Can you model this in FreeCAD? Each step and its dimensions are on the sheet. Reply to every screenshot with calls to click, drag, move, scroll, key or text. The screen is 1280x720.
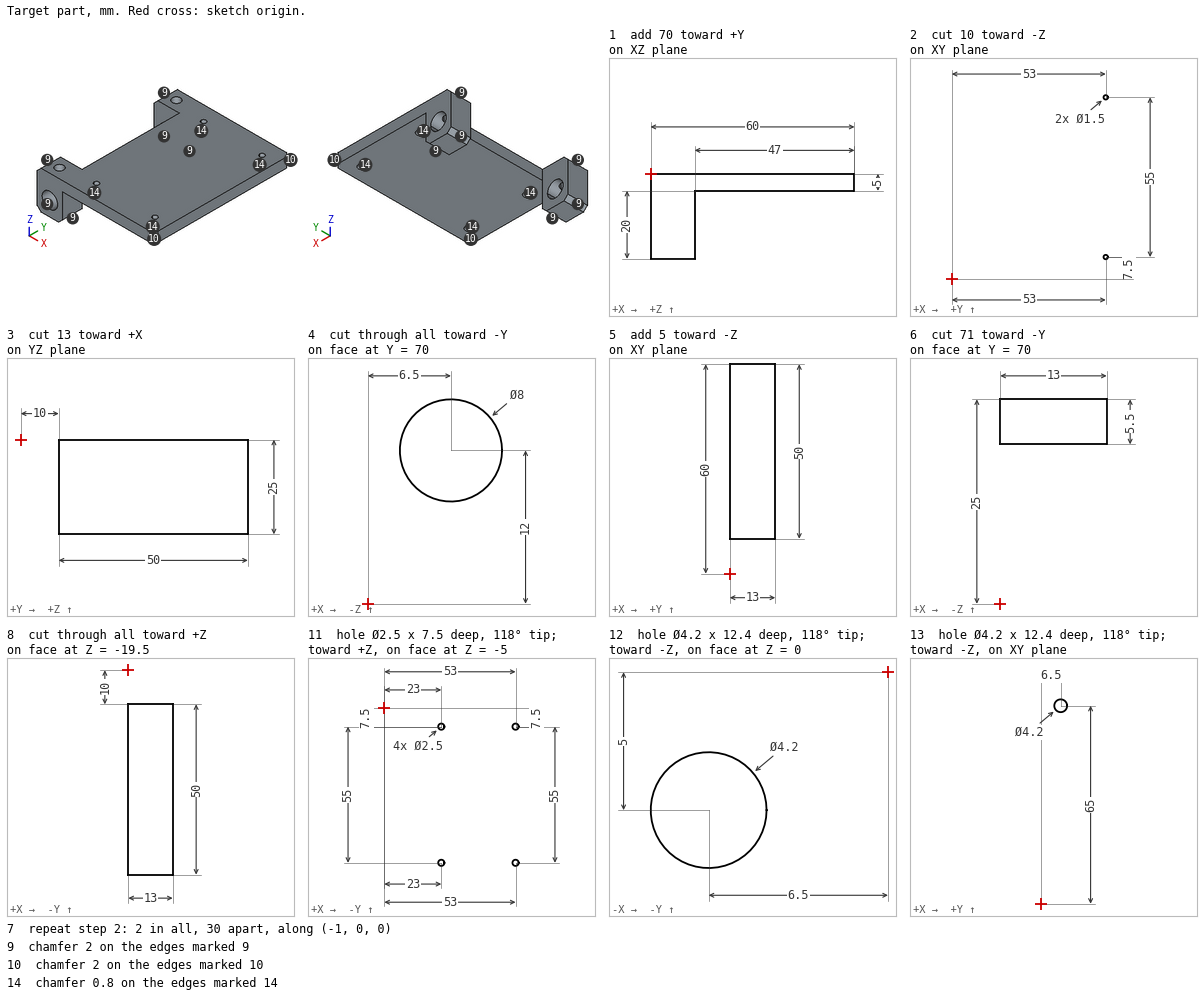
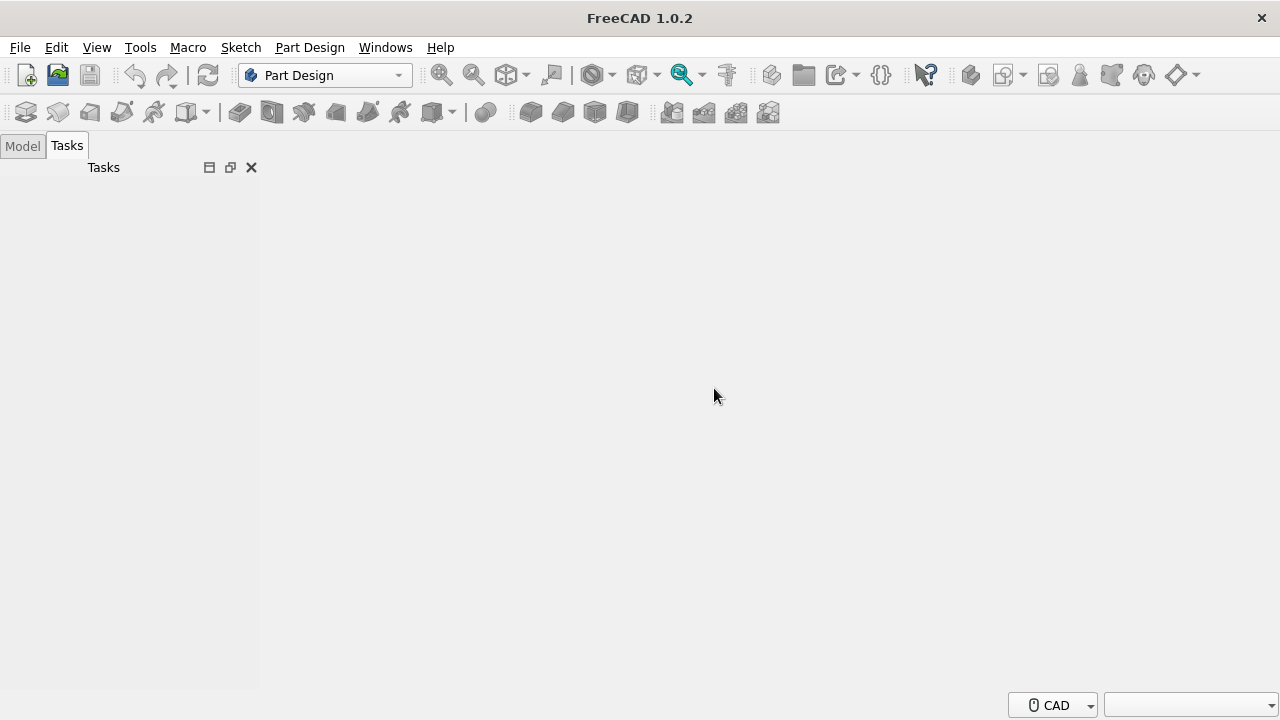
click(26, 76)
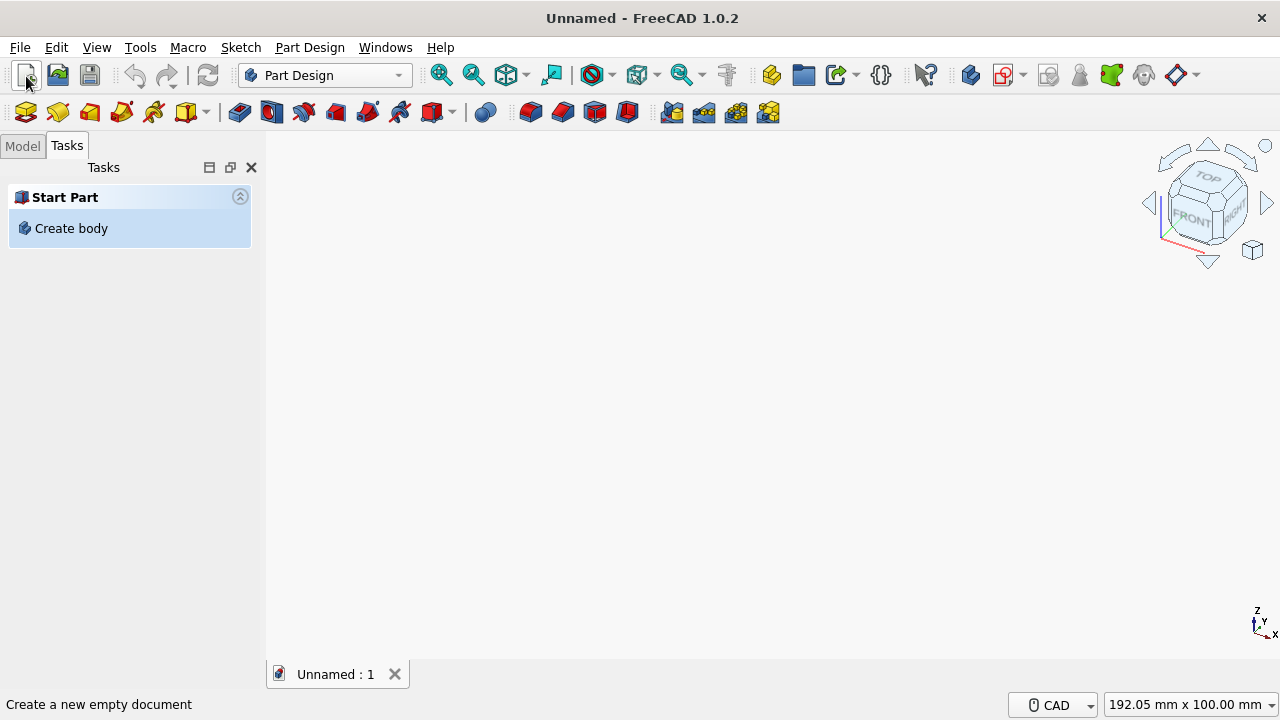
click(1004, 76)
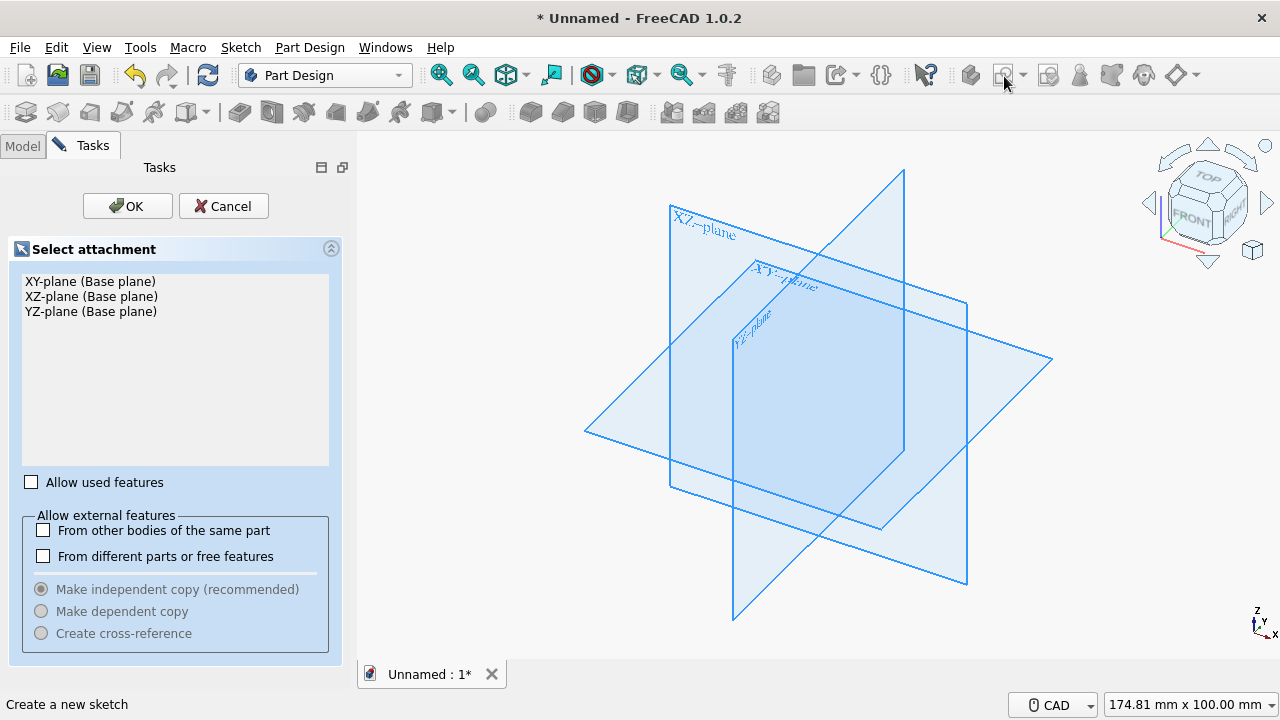
click(82, 296)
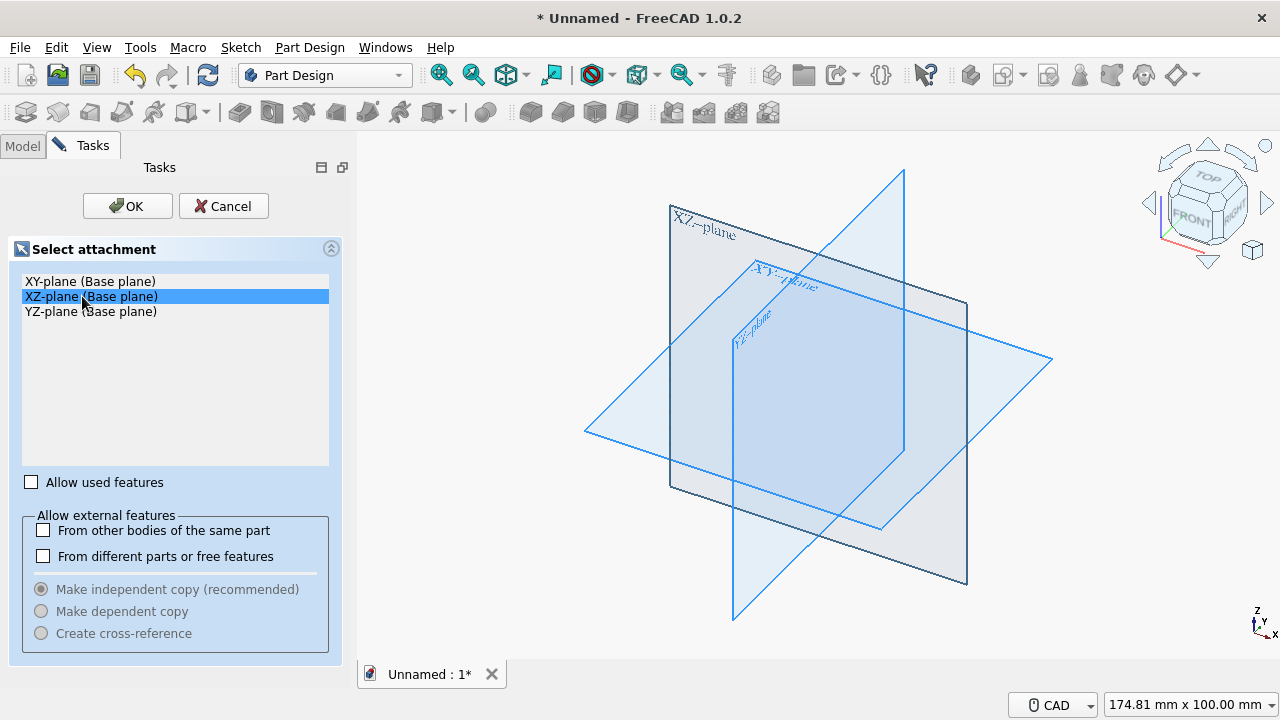
click(128, 206)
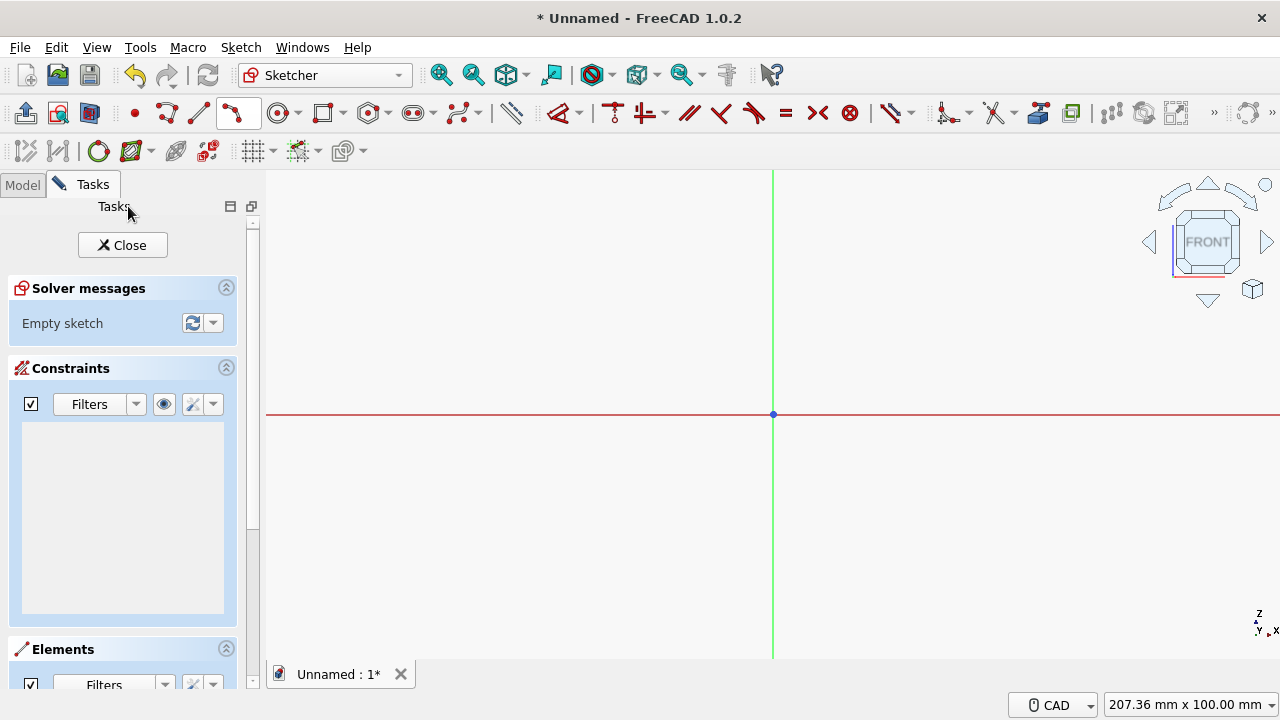
scroll(1115, 550, up, 3)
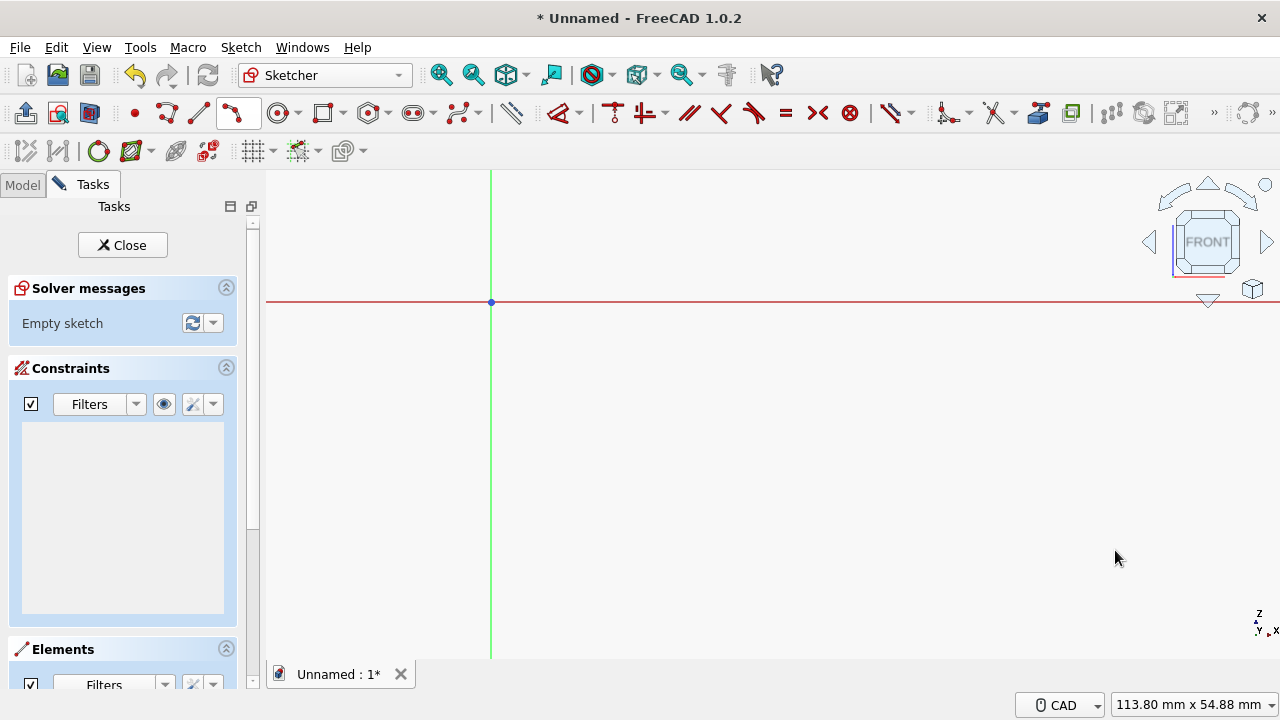
key(g)
key(m)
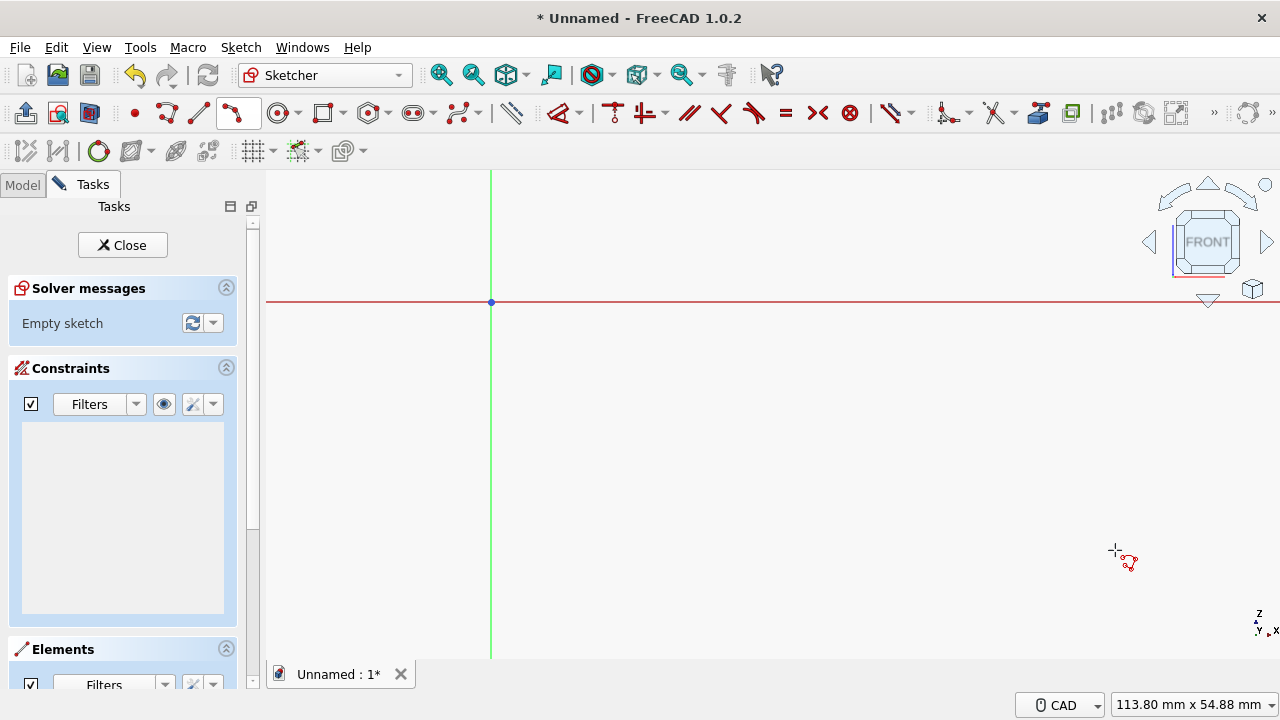
click(491, 302)
click(1026, 311)
click(1026, 347)
click(607, 347)
click(607, 525)
click(500, 525)
click(491, 302)
key(Escape)
key(Escape)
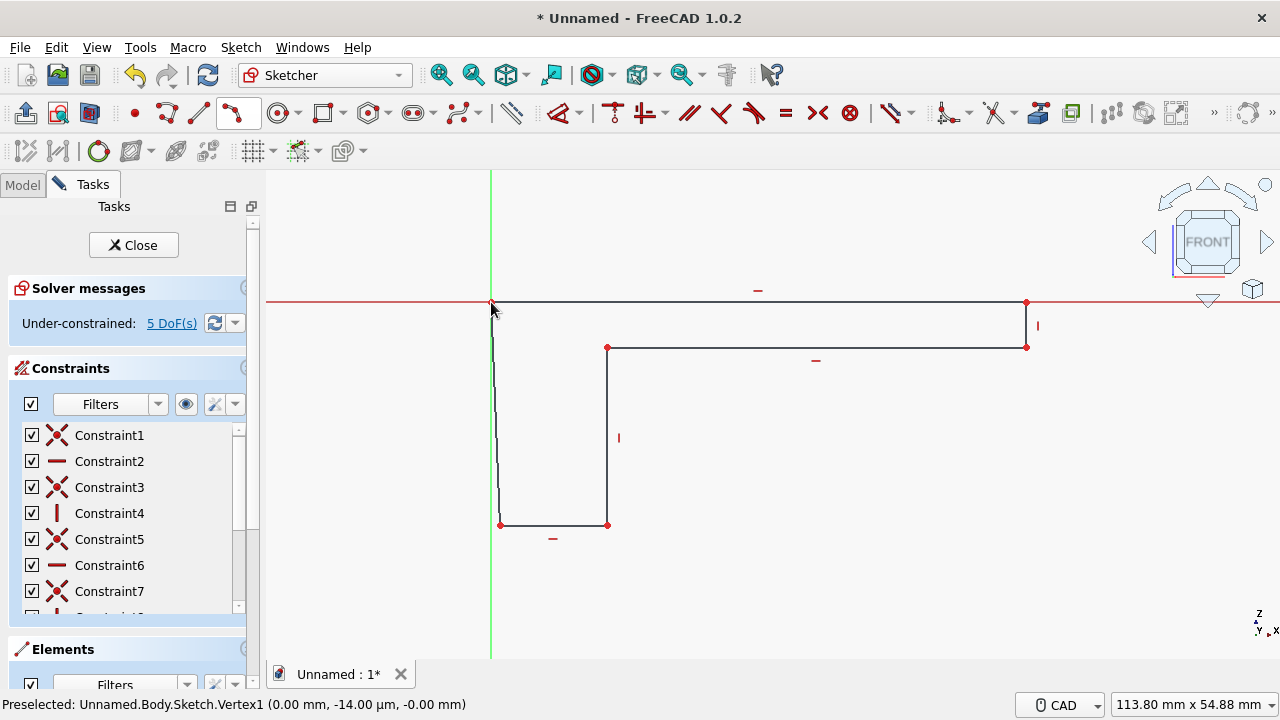
click(494, 370)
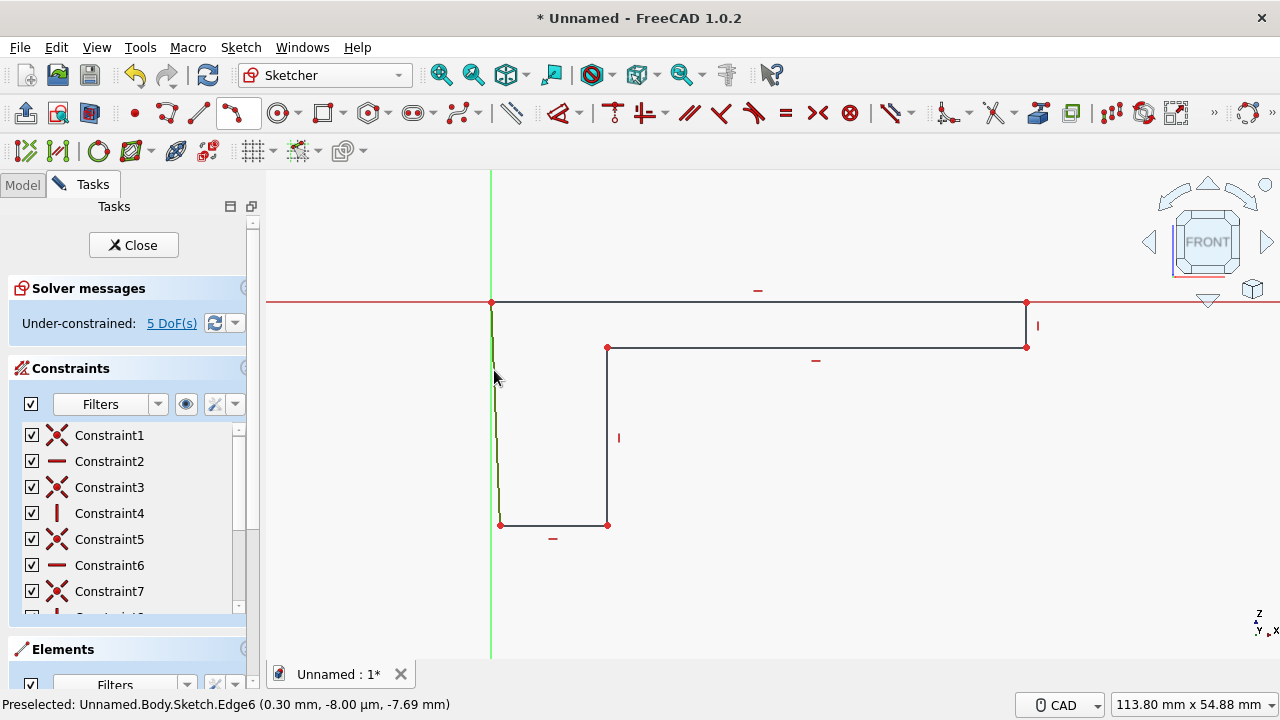
key(v)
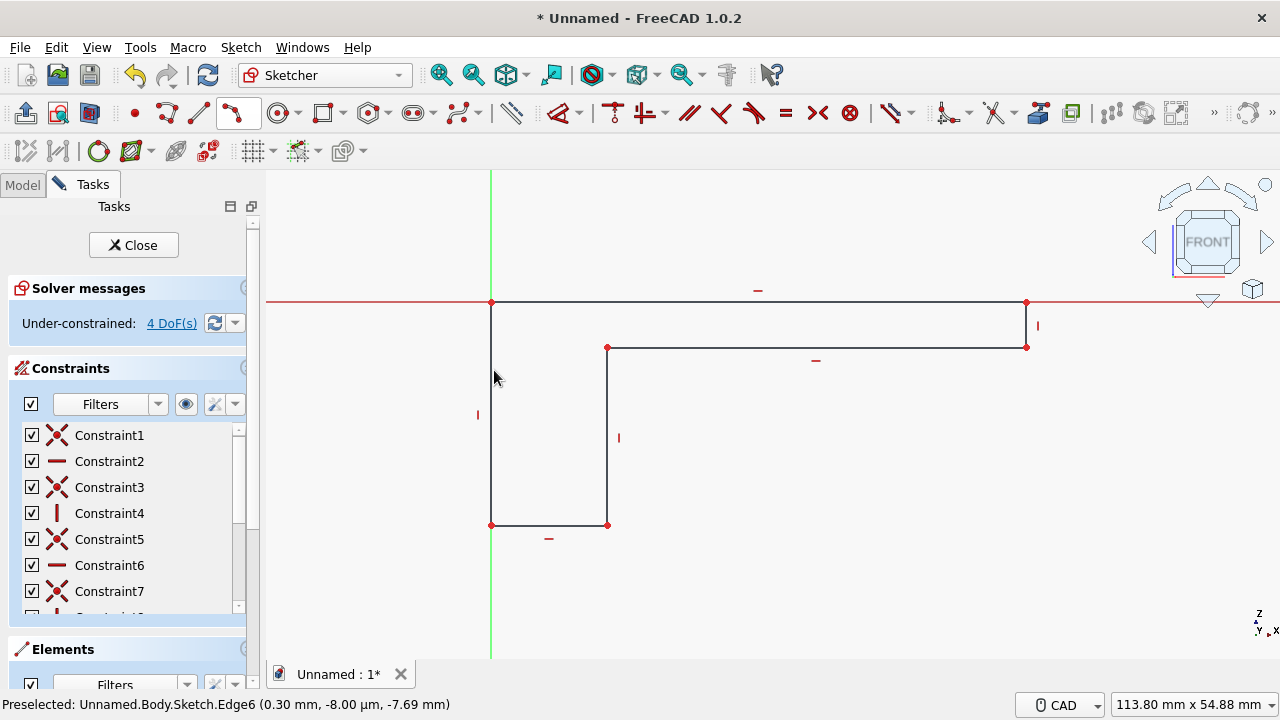
click(558, 114)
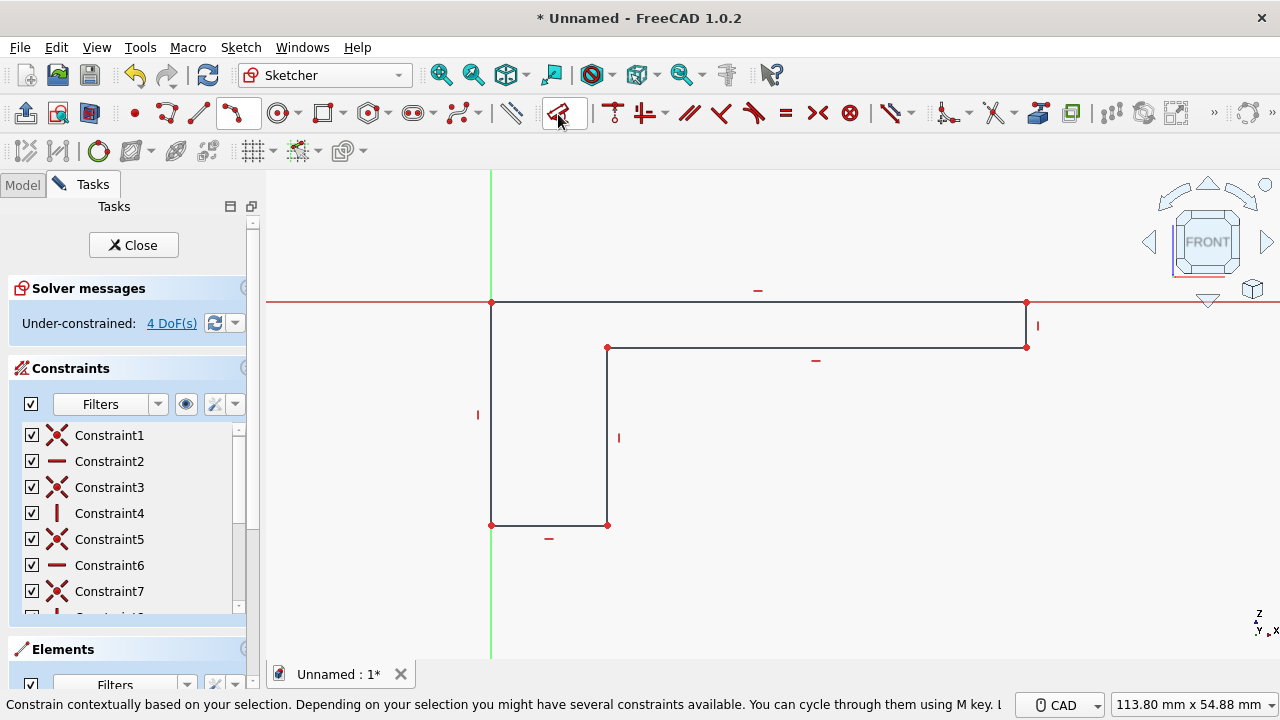
click(1026, 316)
click(1060, 325)